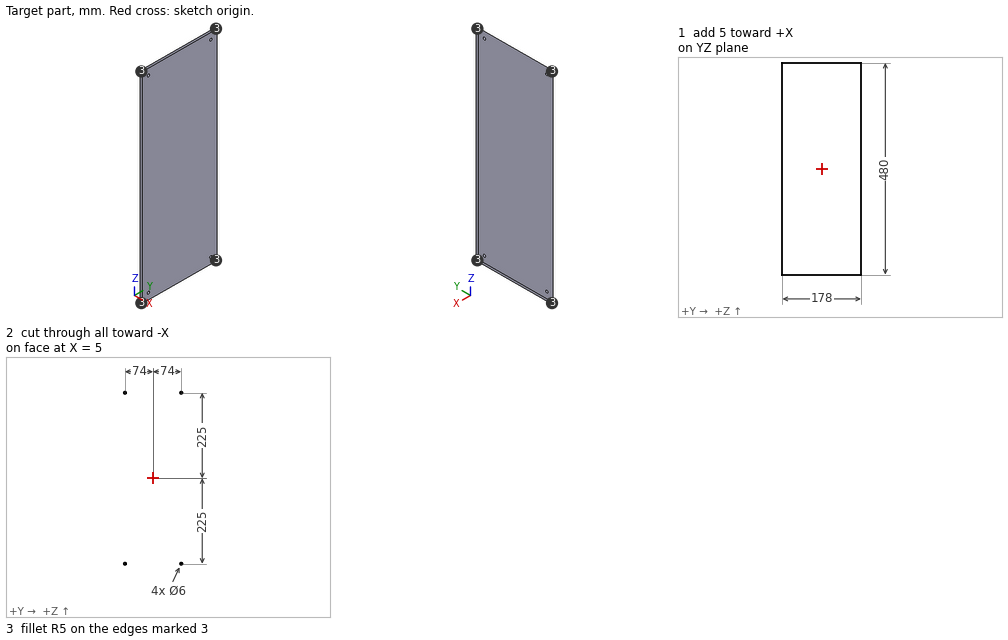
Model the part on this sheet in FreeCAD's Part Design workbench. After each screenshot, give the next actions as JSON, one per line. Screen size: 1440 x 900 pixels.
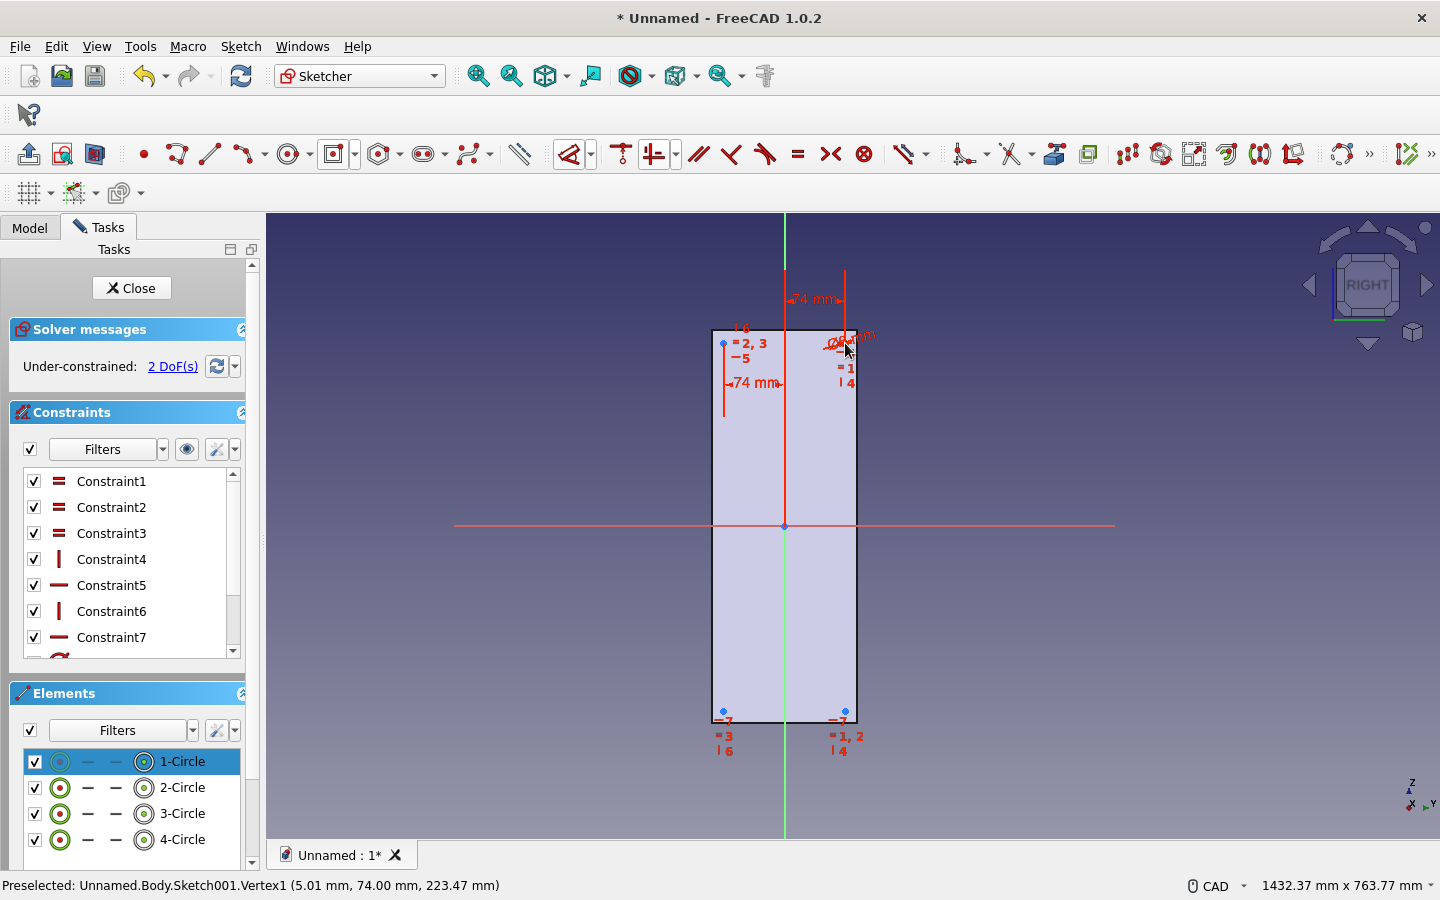
{"action": "left_click", "coordinate": [590, 154]}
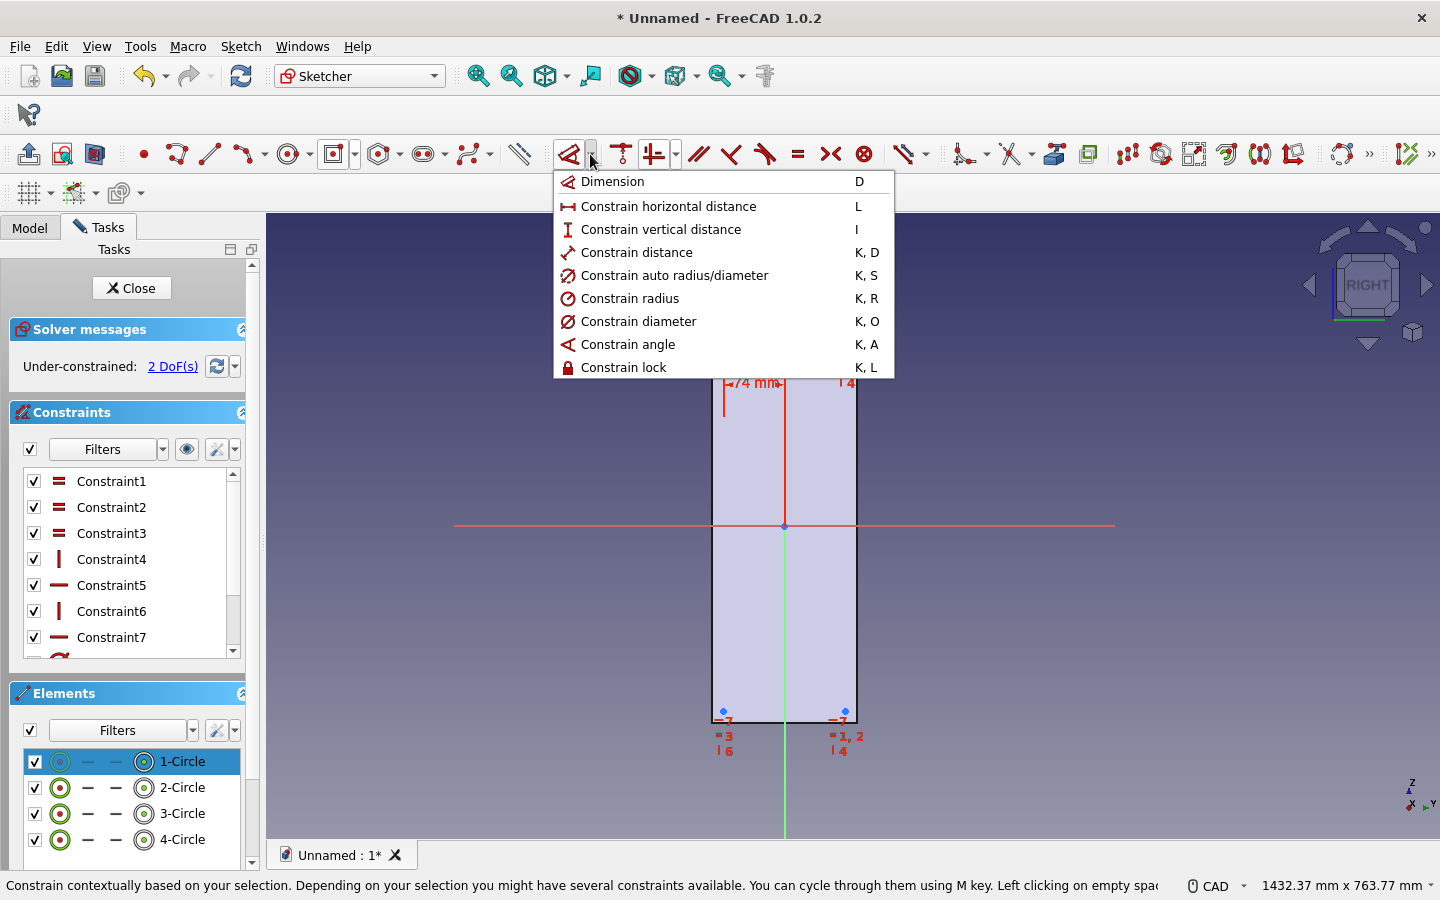
{"action": "left_click", "coordinate": [724, 230]}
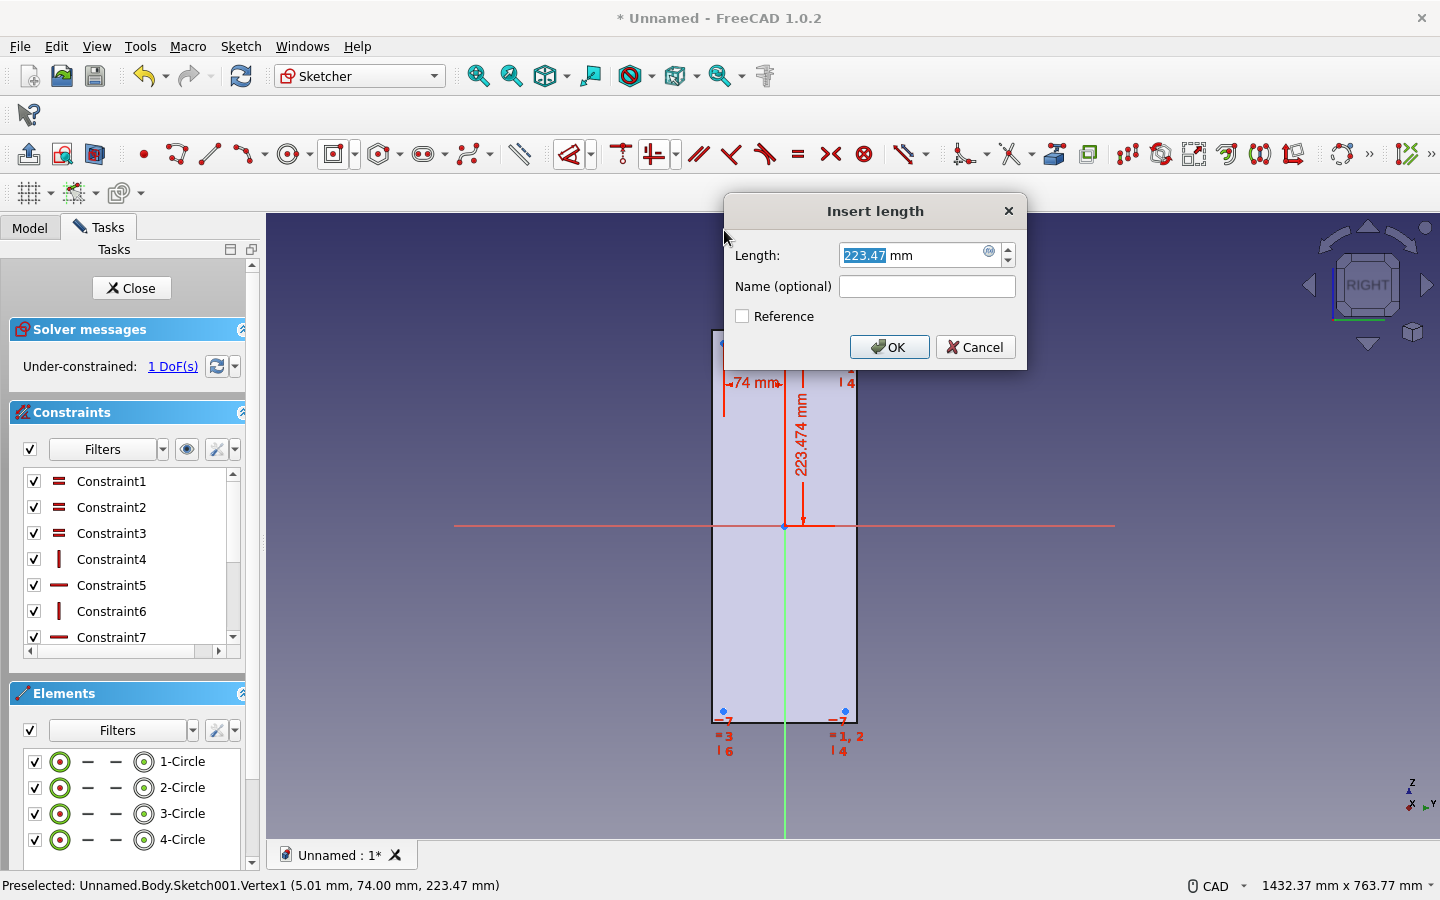
{"action": "type", "text": "225"}
{"action": "key", "text": "Return"}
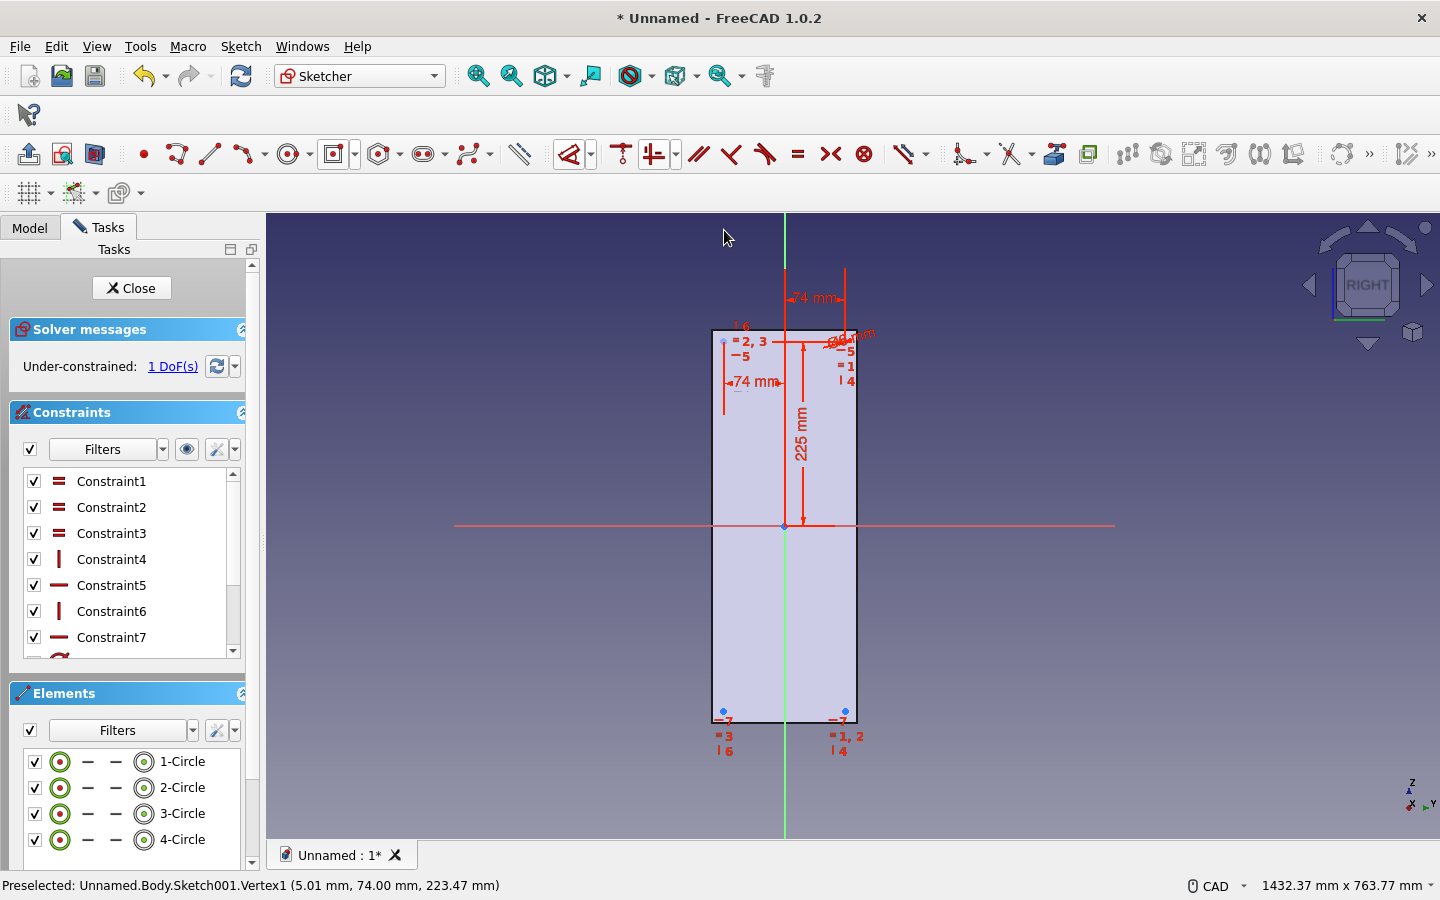
{"action": "left_click", "coordinate": [845, 711]}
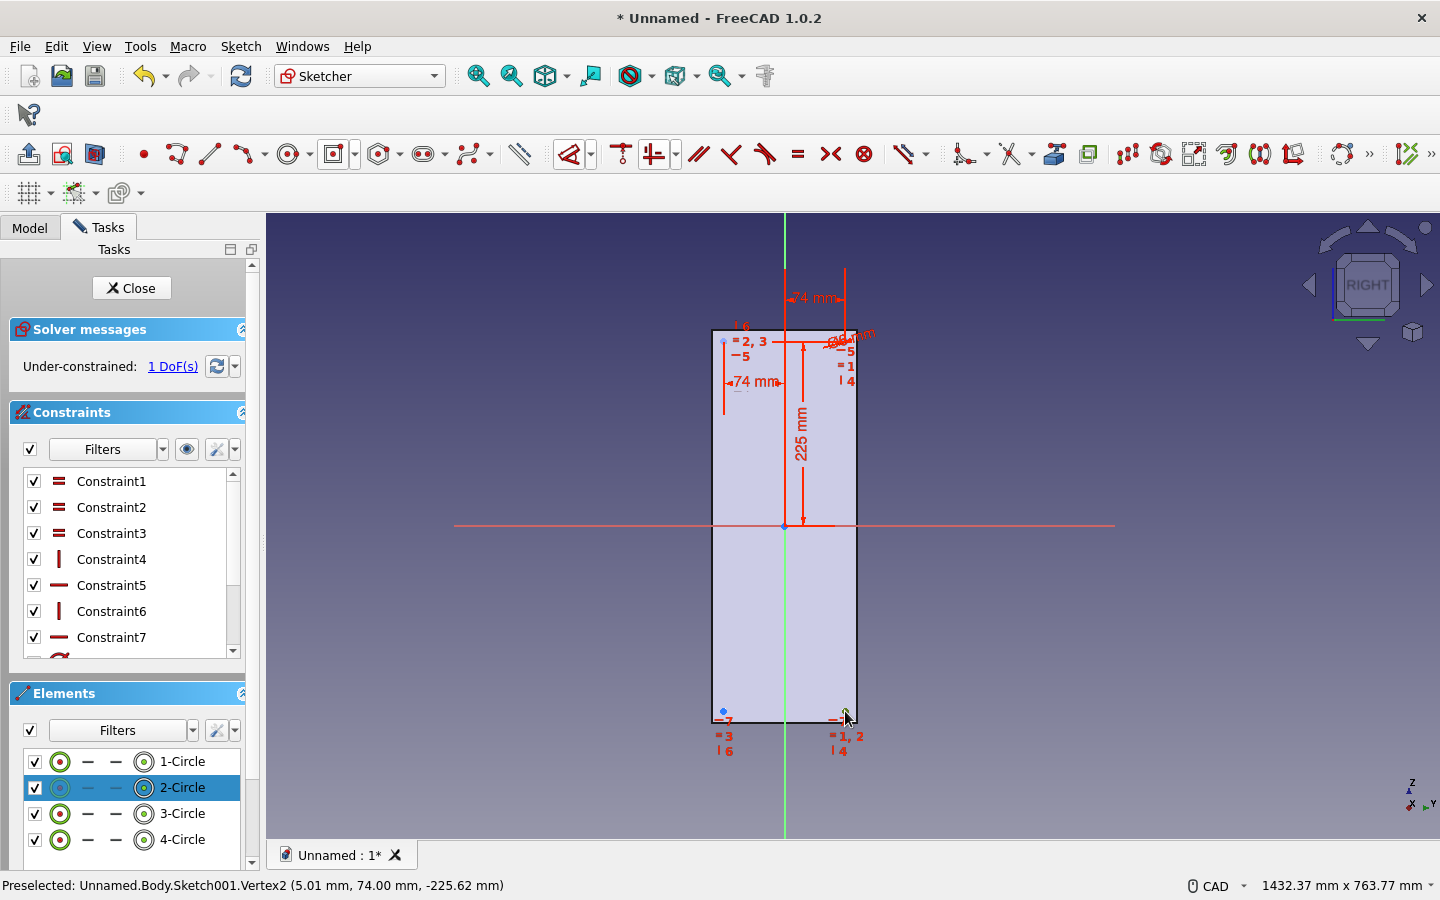
{"action": "left_click", "coordinate": [590, 154]}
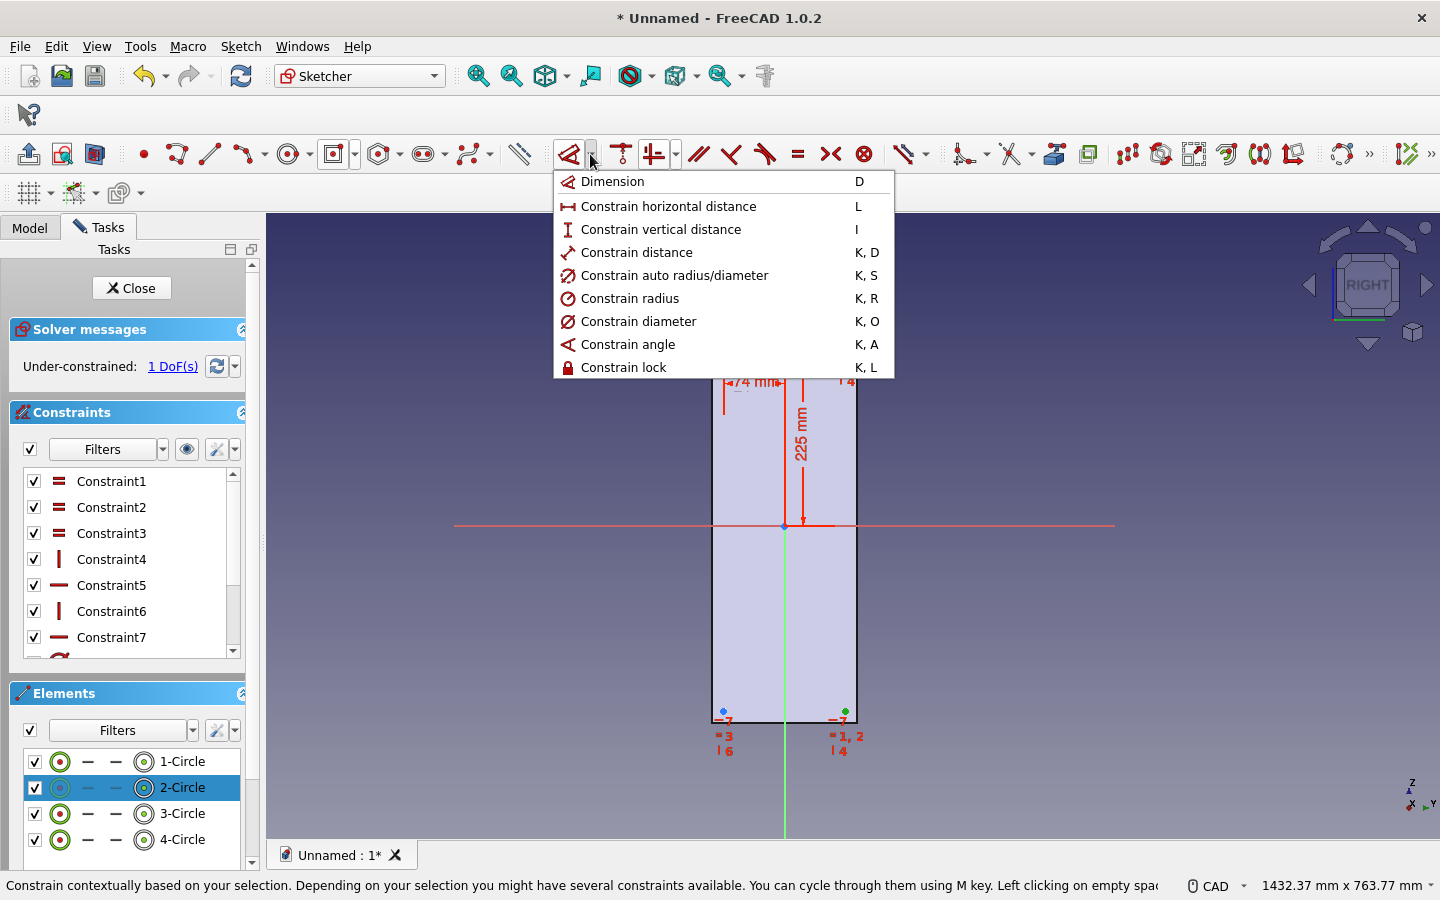
{"action": "left_click", "coordinate": [724, 230]}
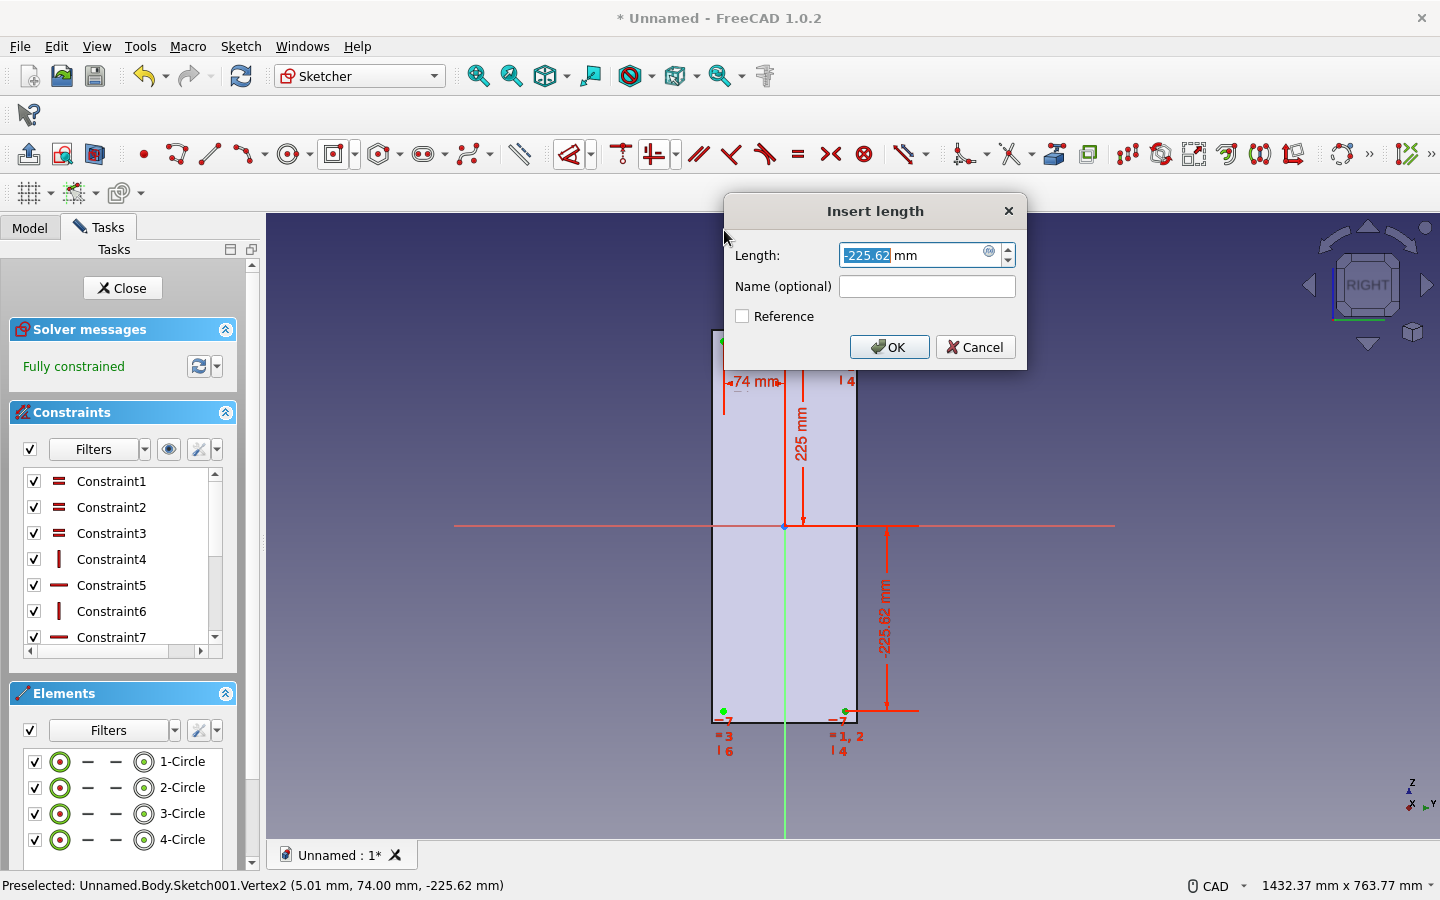
{"action": "type", "text": "-225"}
{"action": "key", "text": "Return"}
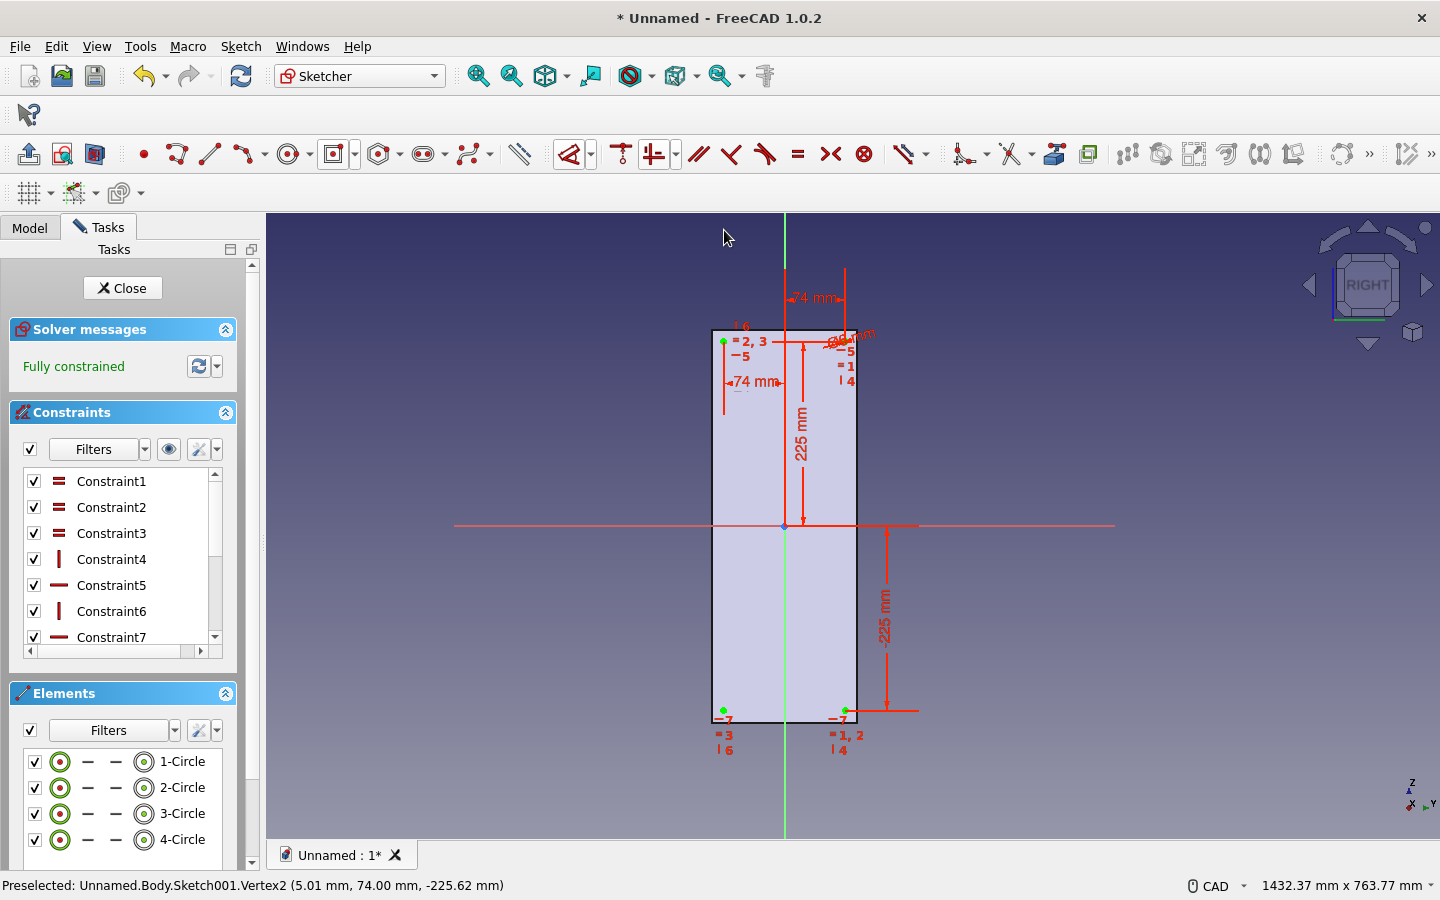
{"action": "left_click", "coordinate": [123, 288]}